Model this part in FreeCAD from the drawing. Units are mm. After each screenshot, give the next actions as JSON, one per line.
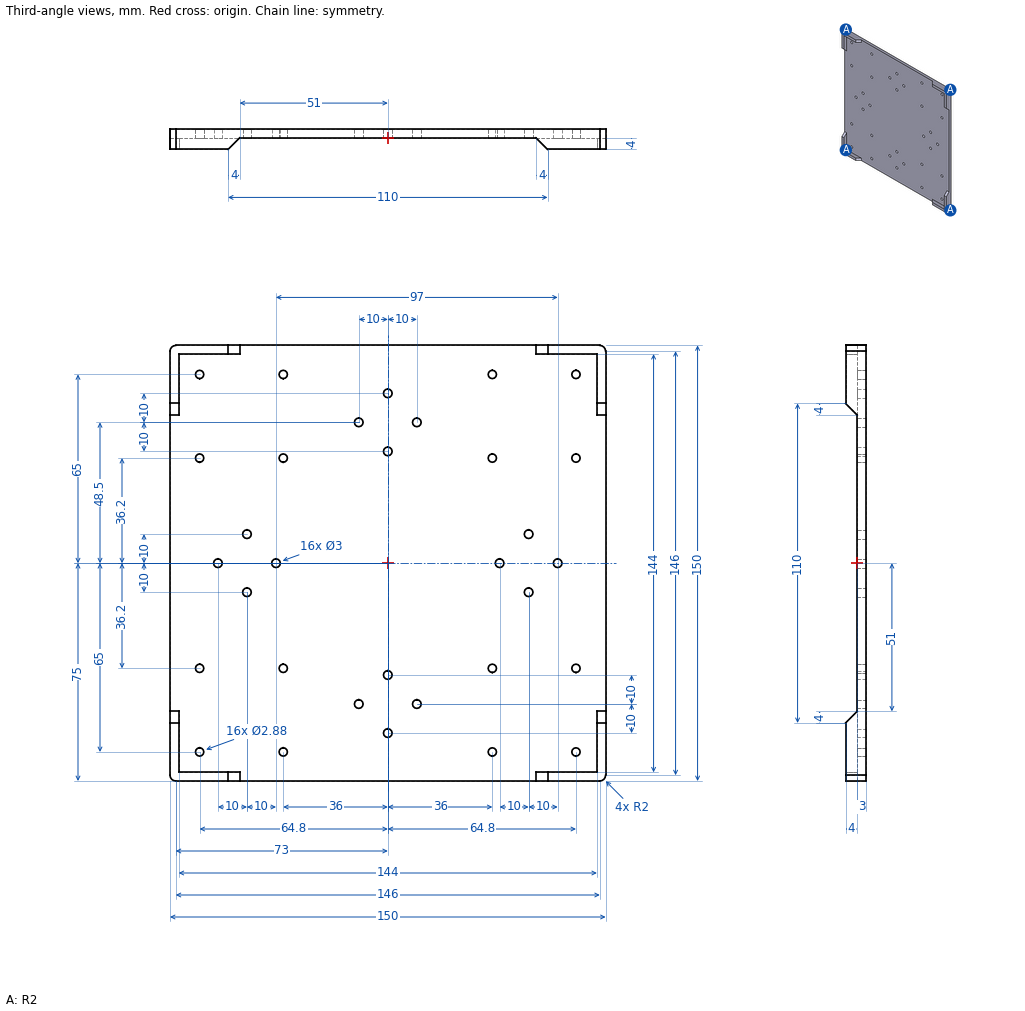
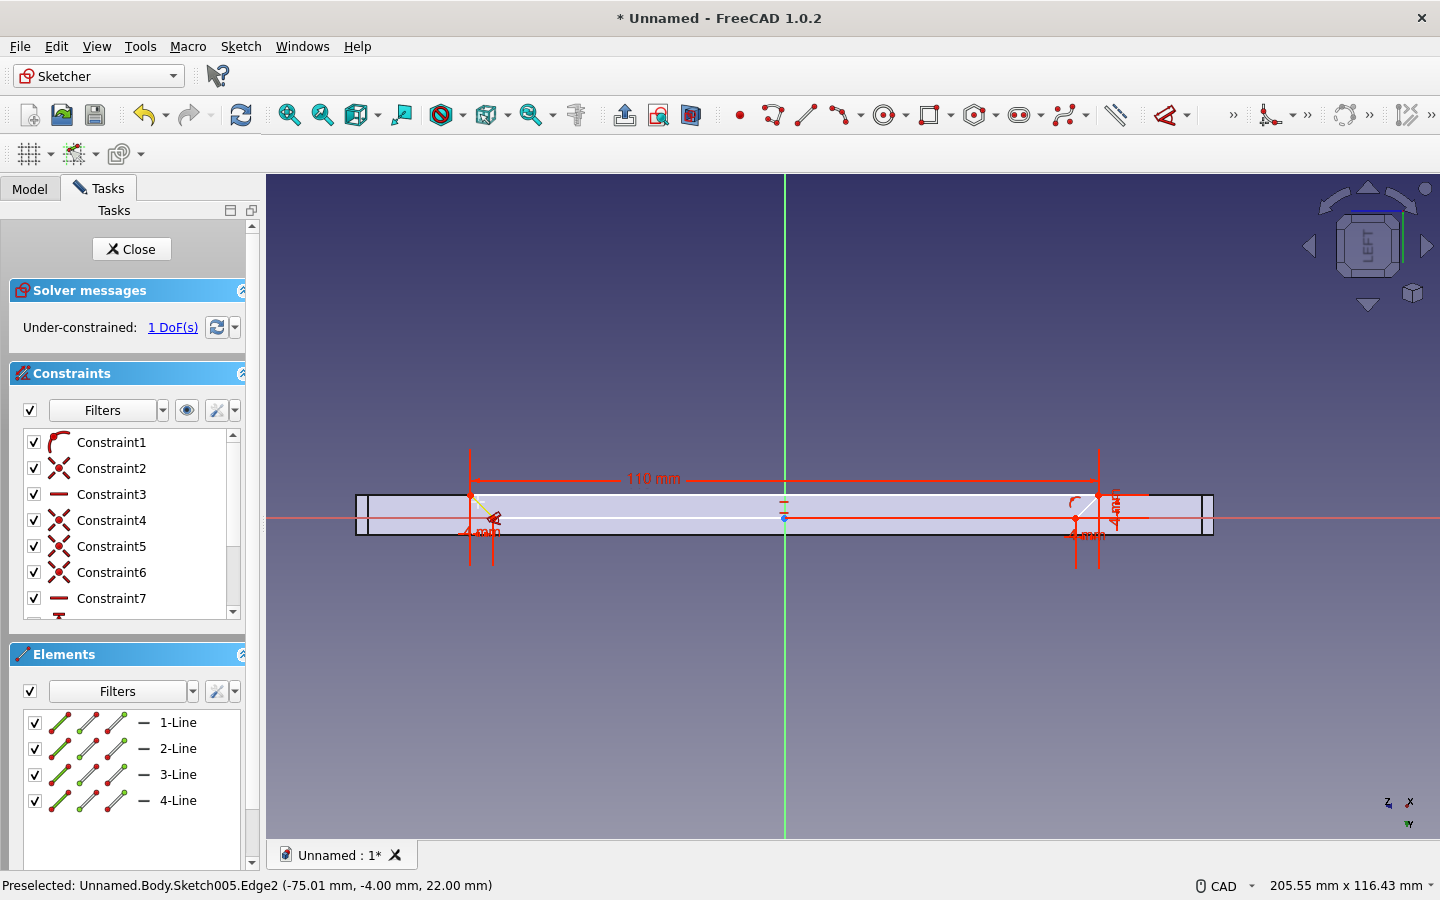
{"action": "left_click", "coordinate": [1076, 518]}
{"action": "left_click", "coordinate": [930, 552]}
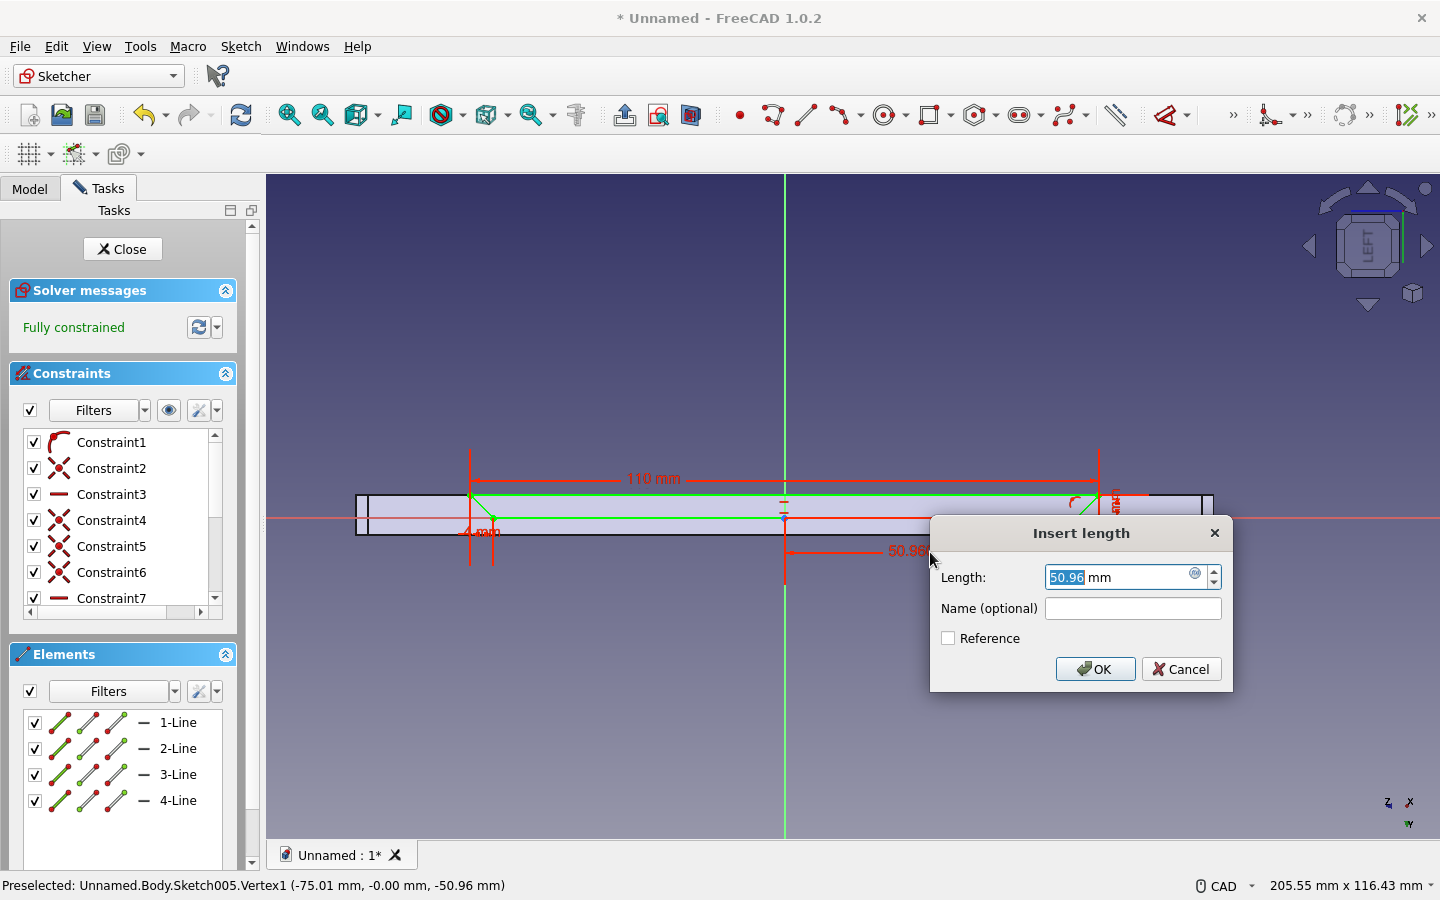
{"action": "type", "text": "51"}
{"action": "key", "text": "Return"}
{"action": "key", "text": "Escape"}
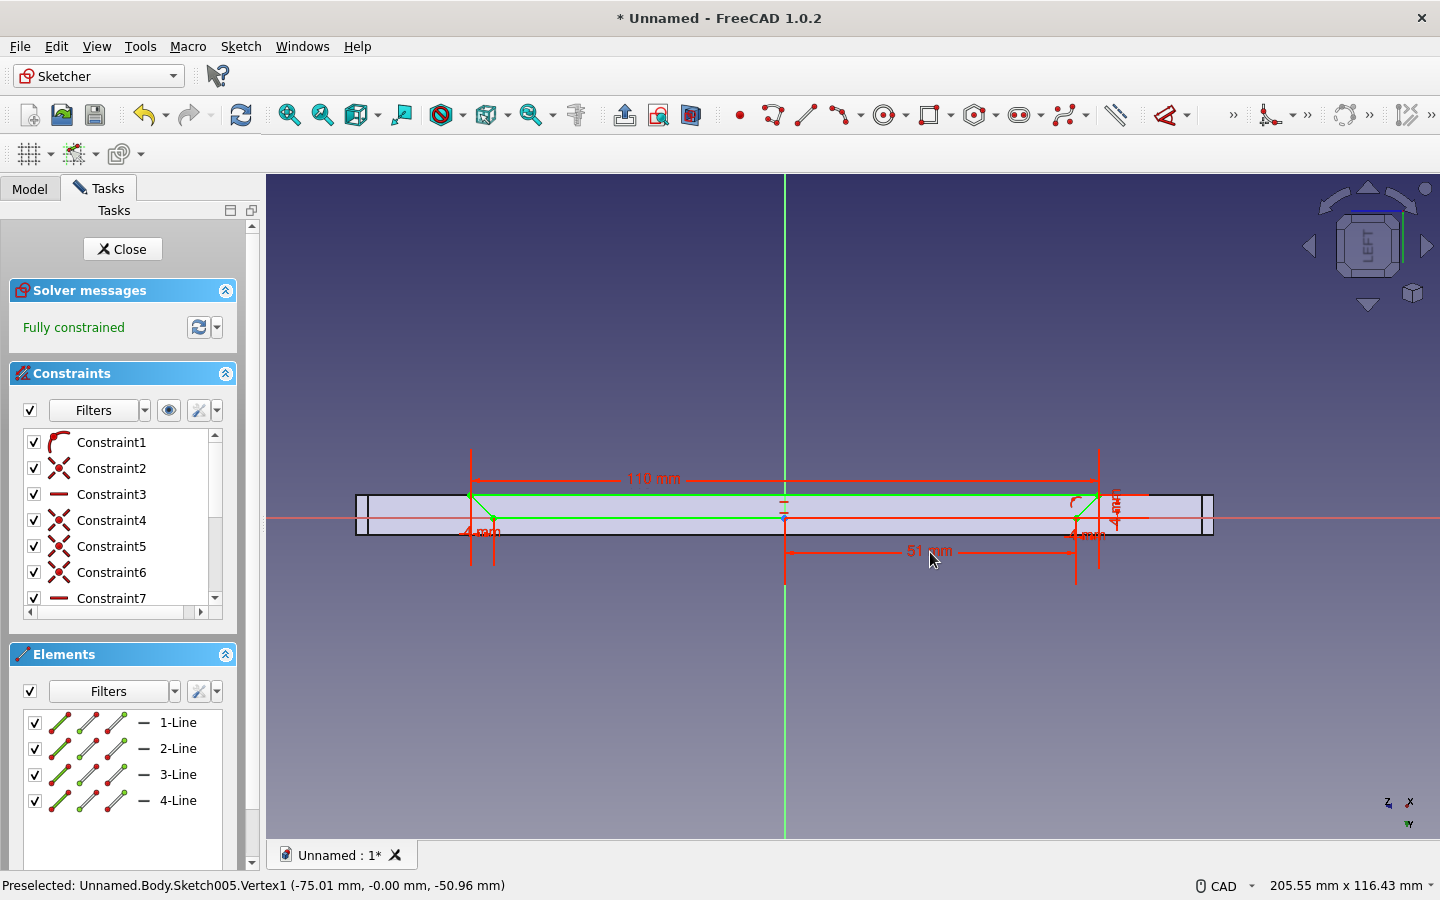
{"action": "left_click", "coordinate": [123, 249]}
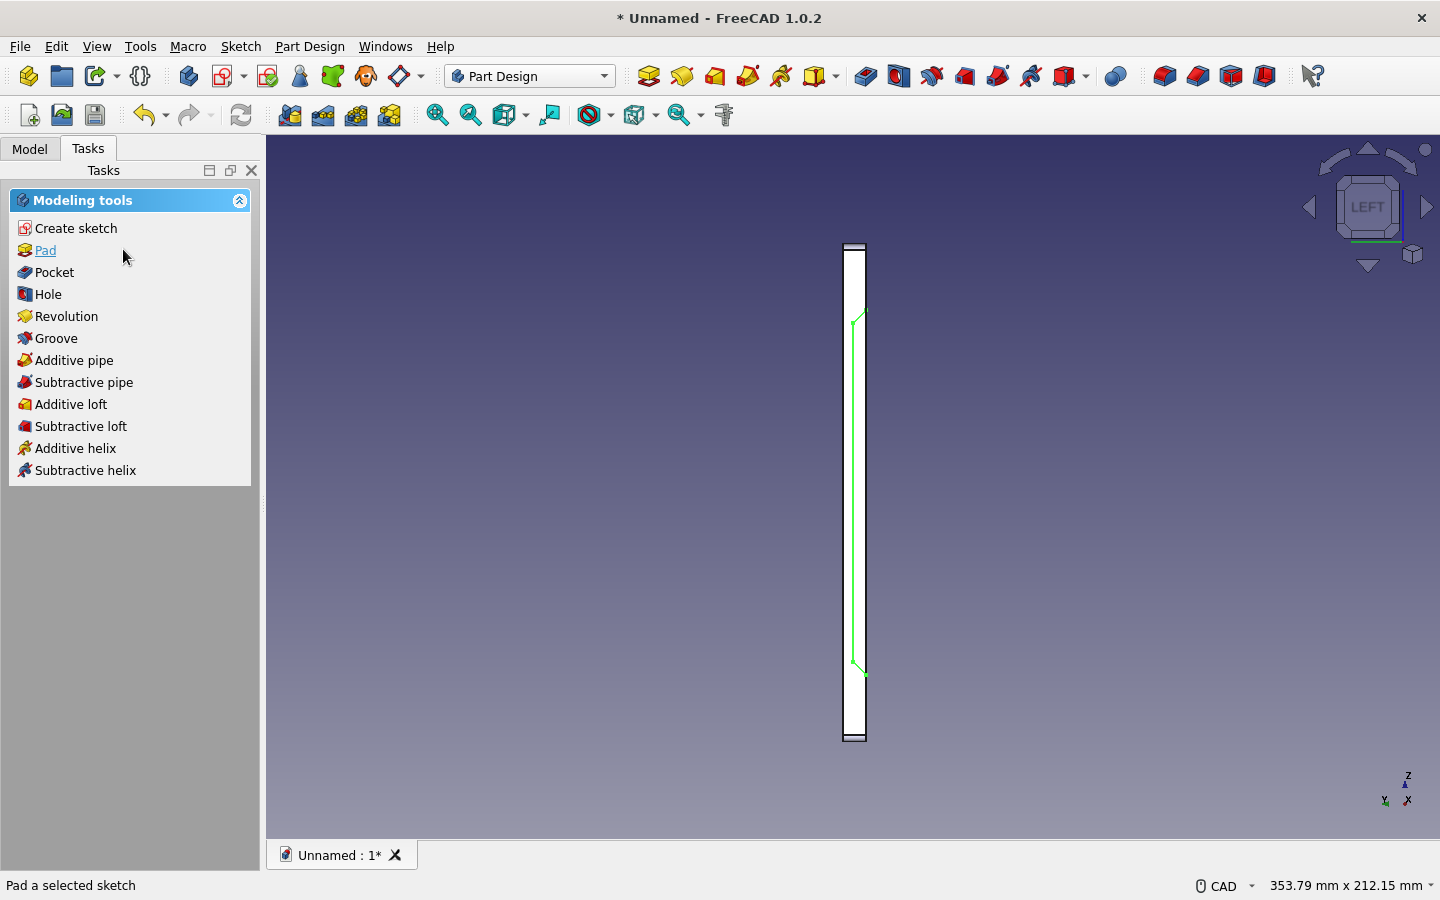
{"action": "left_click", "coordinate": [866, 76]}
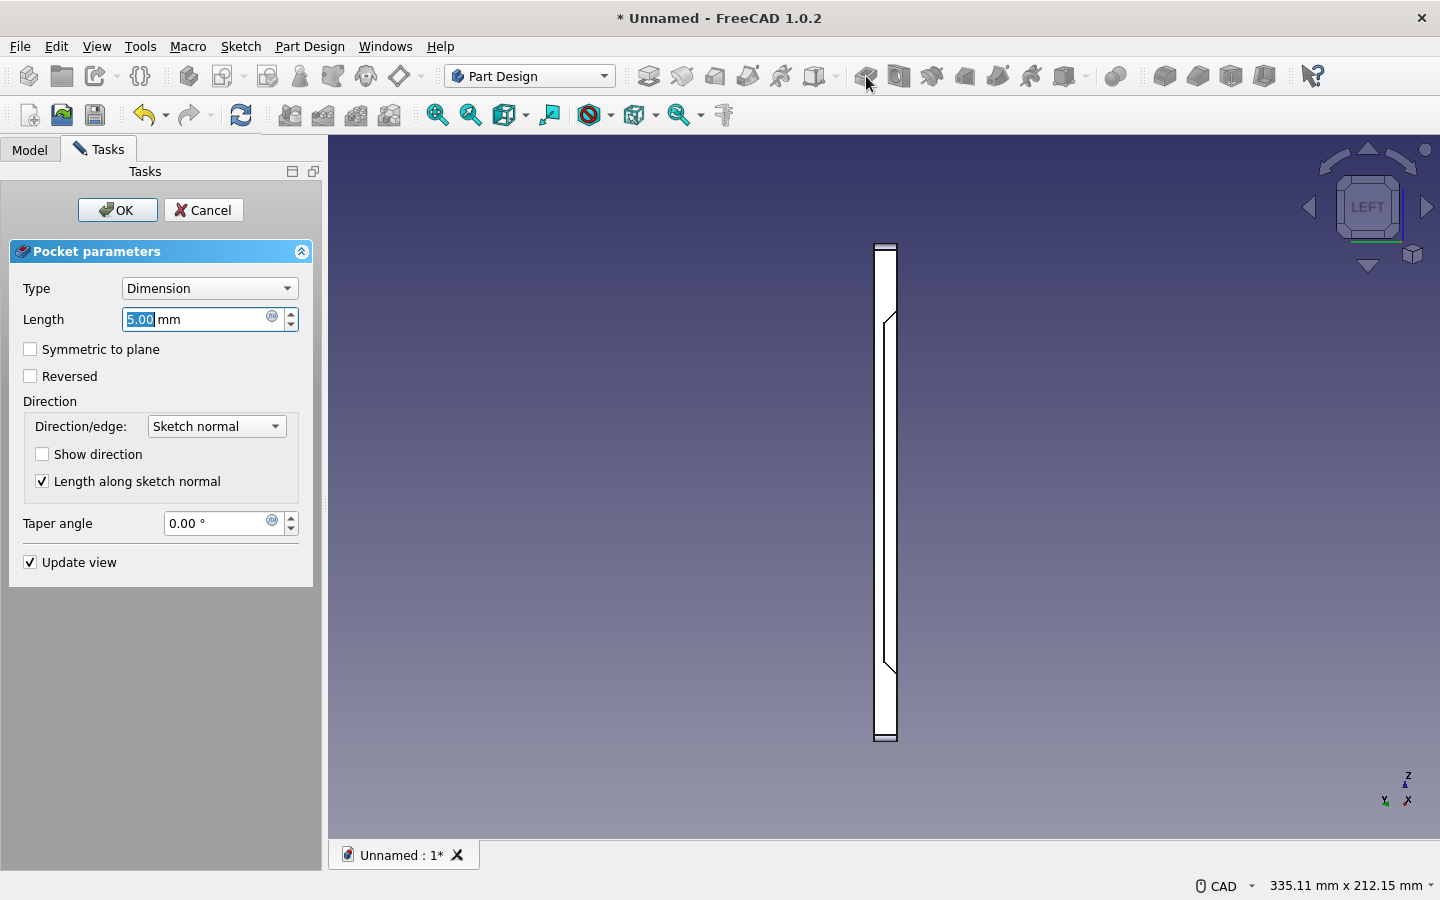
{"action": "left_click", "coordinate": [210, 288]}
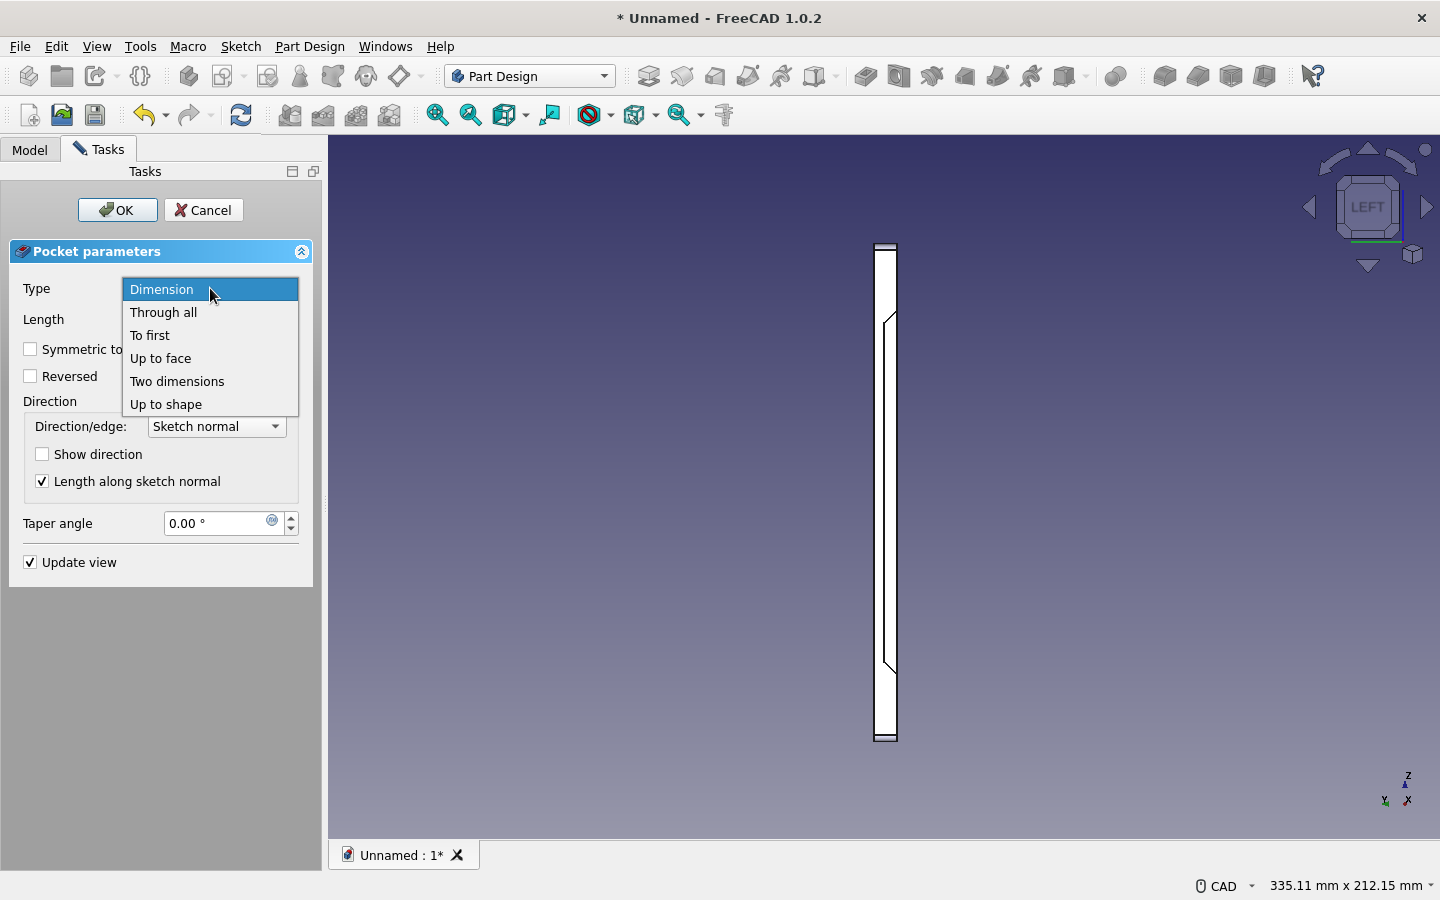
{"action": "left_click", "coordinate": [208, 312]}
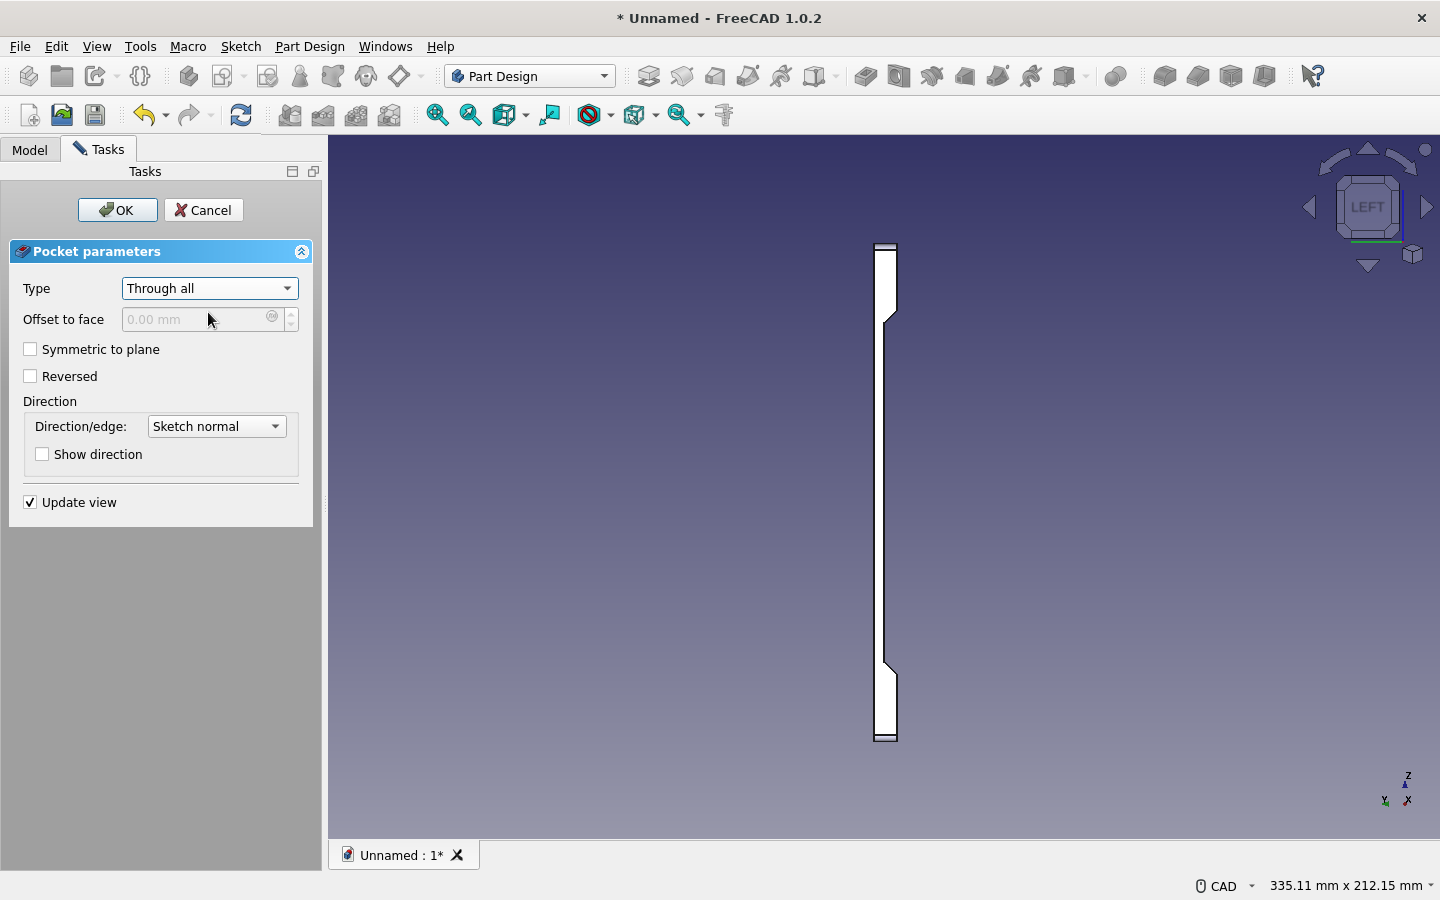
{"action": "left_click", "coordinate": [118, 210]}